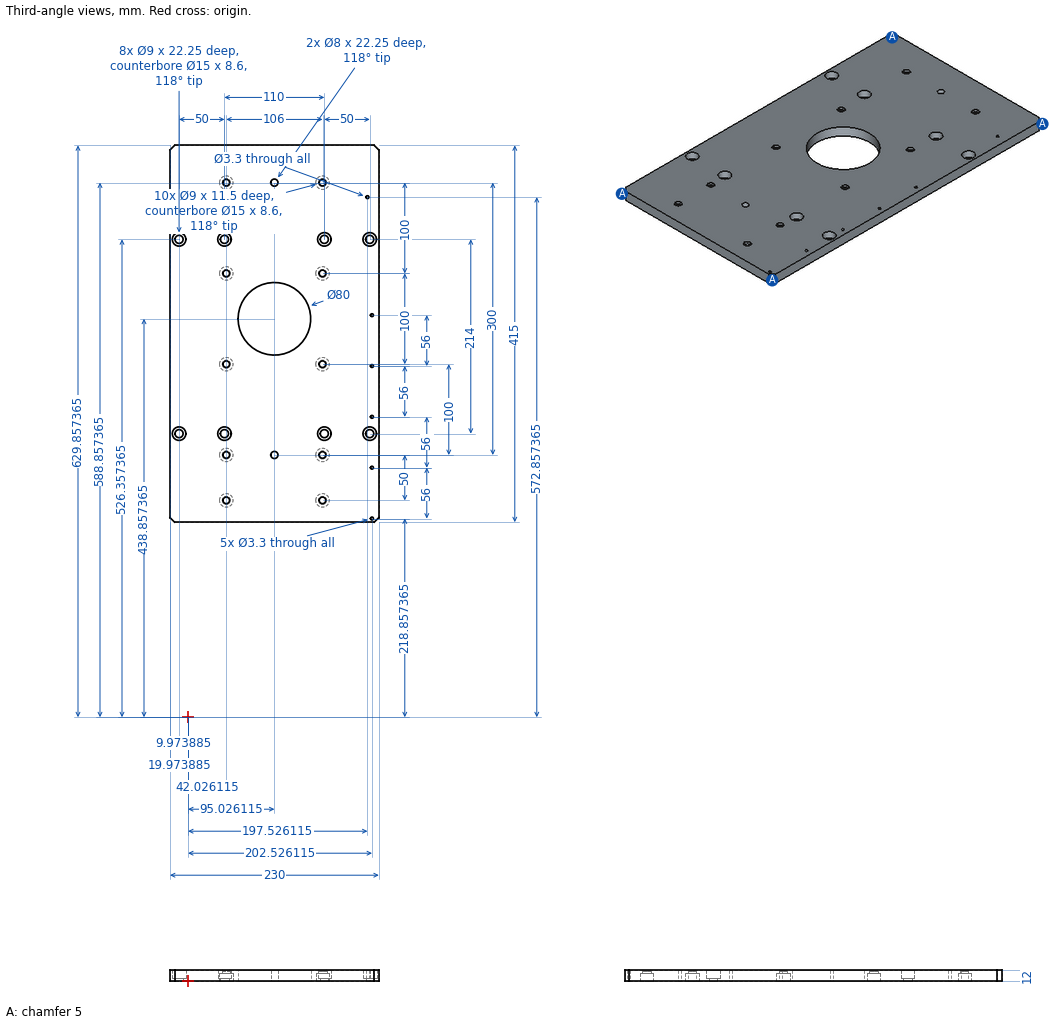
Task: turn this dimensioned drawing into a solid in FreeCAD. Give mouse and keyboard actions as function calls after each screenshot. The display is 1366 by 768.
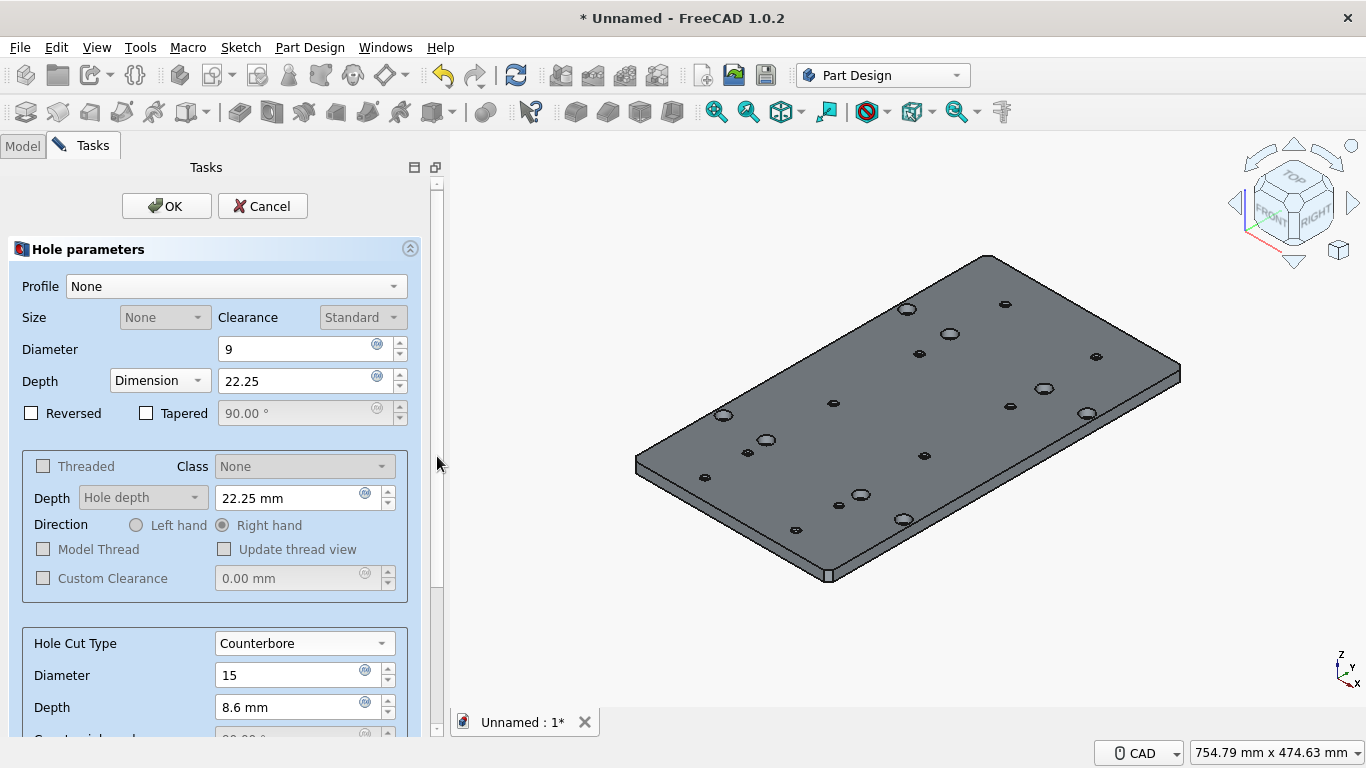
click(167, 206)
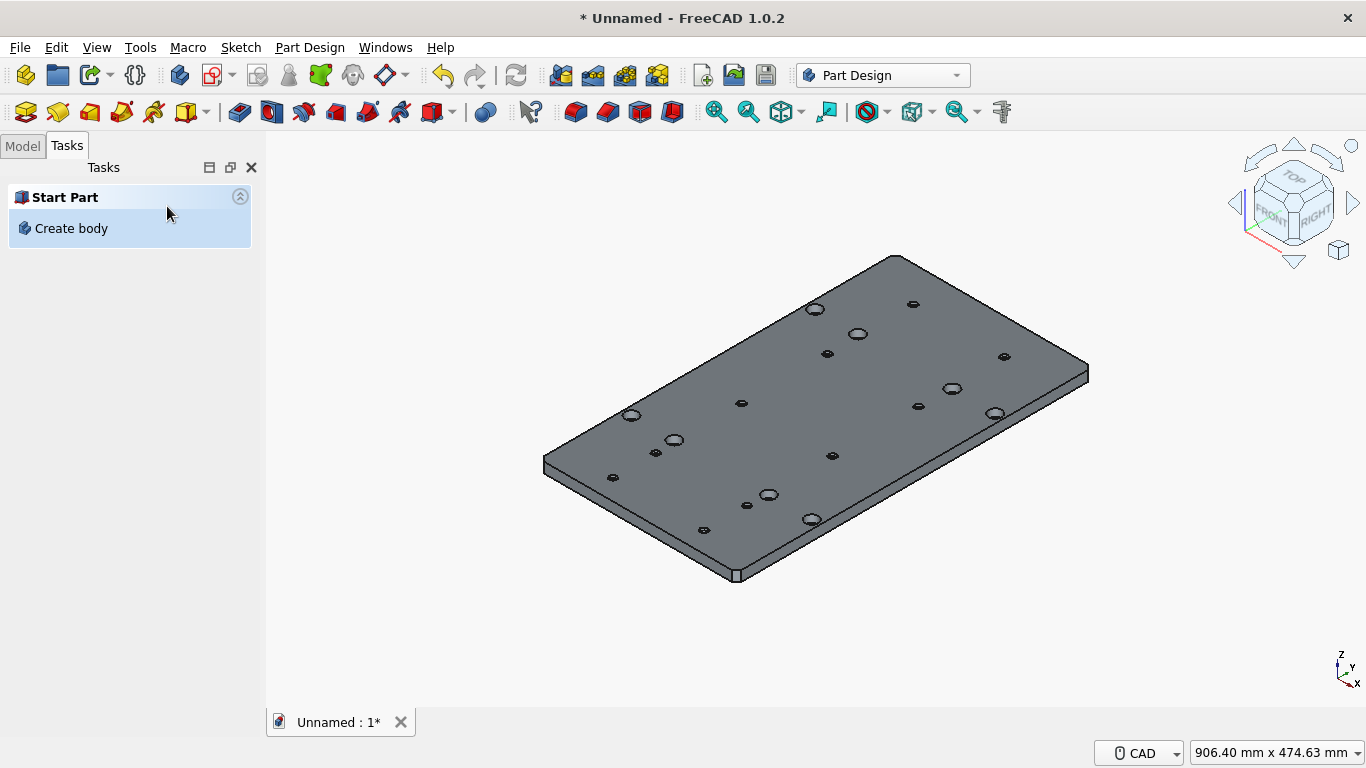
click(816, 412)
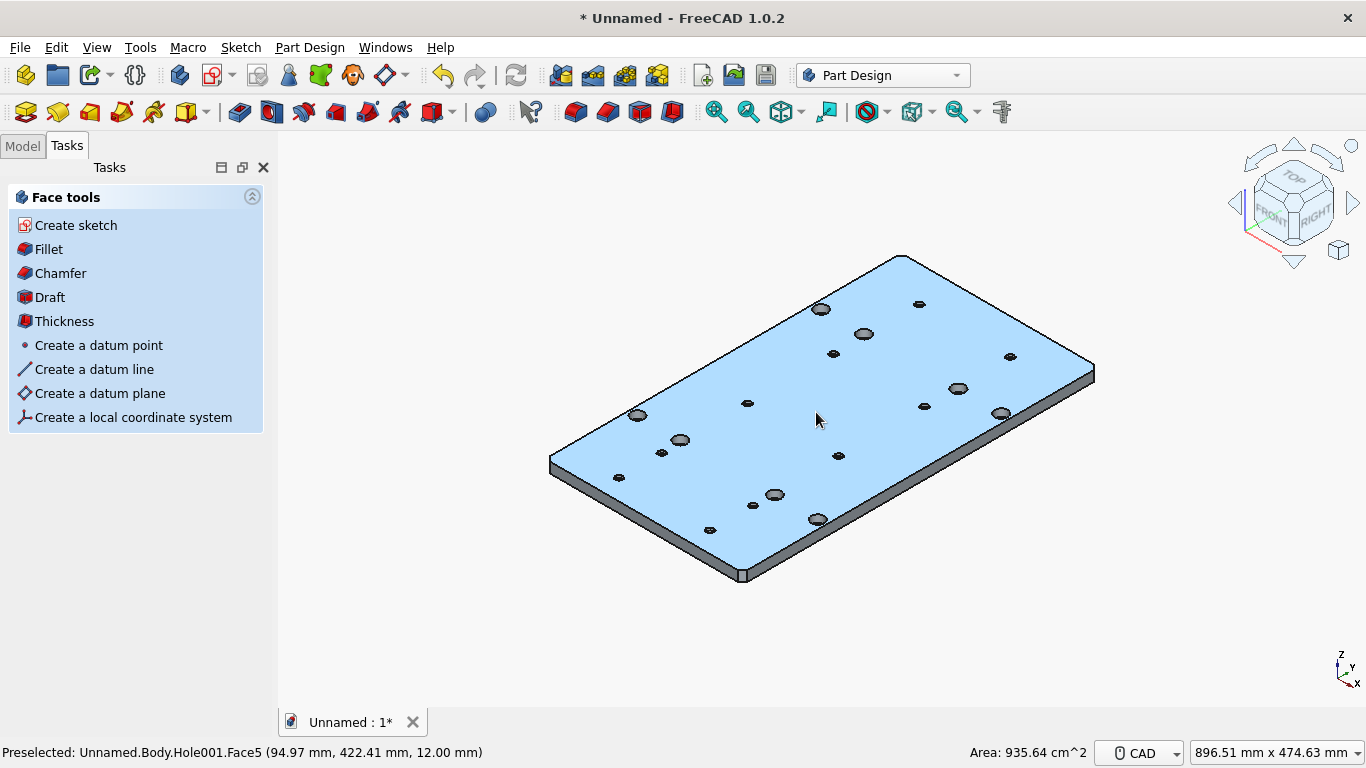
click(212, 76)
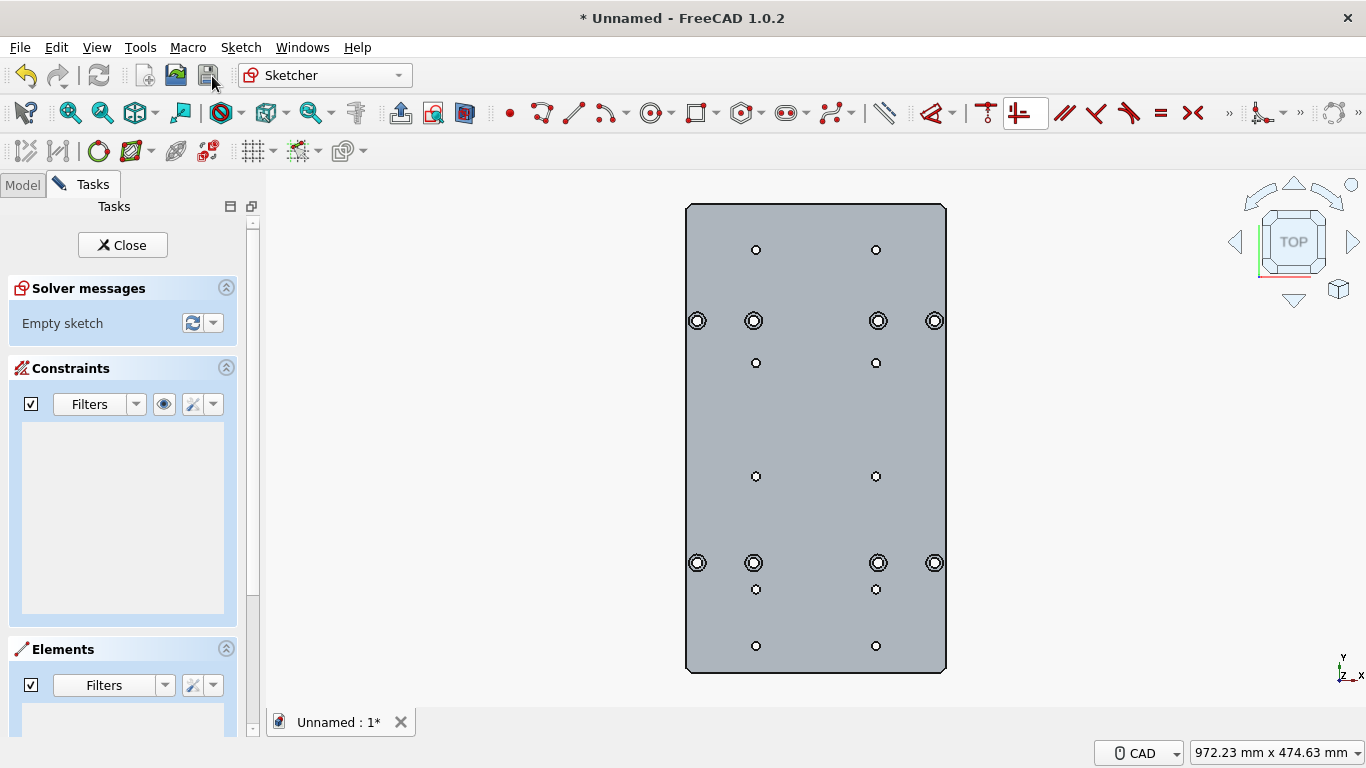
scroll(727, 265, down, 3)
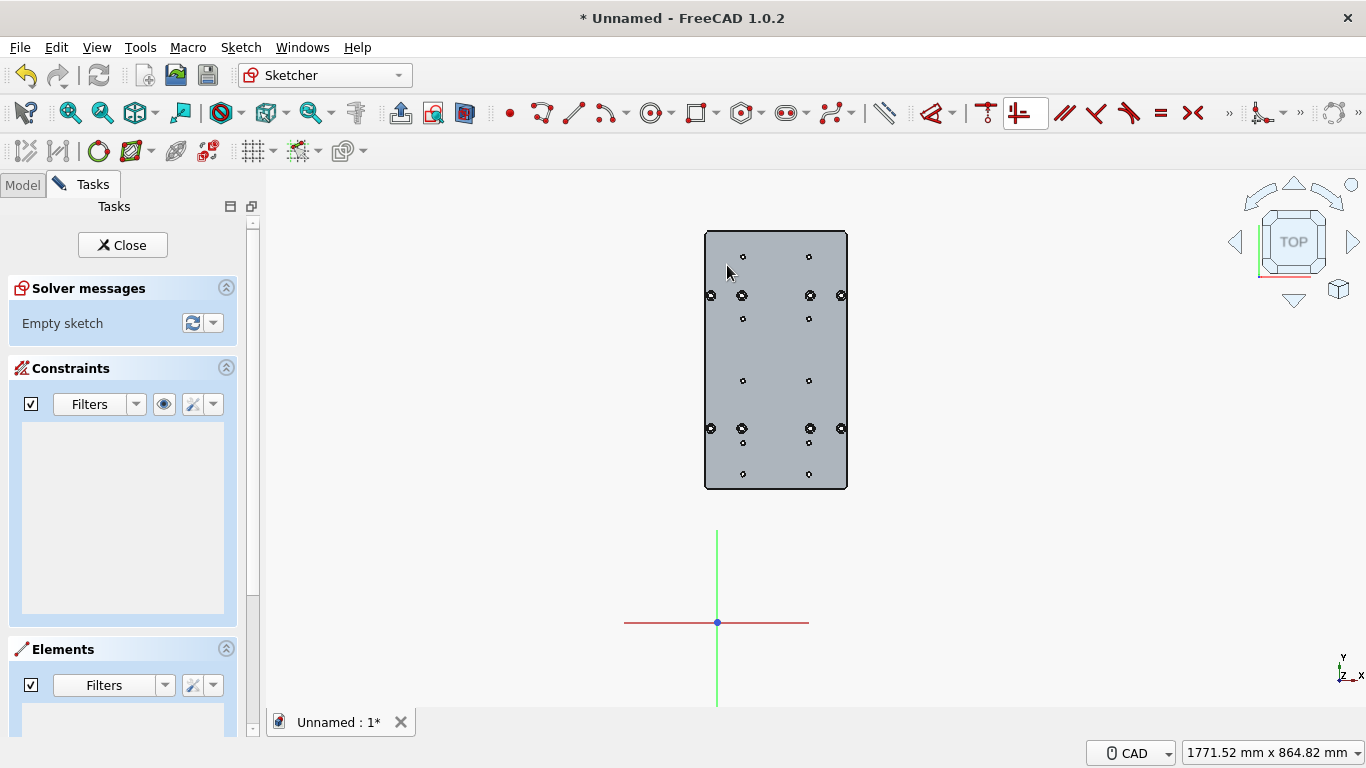
click(652, 114)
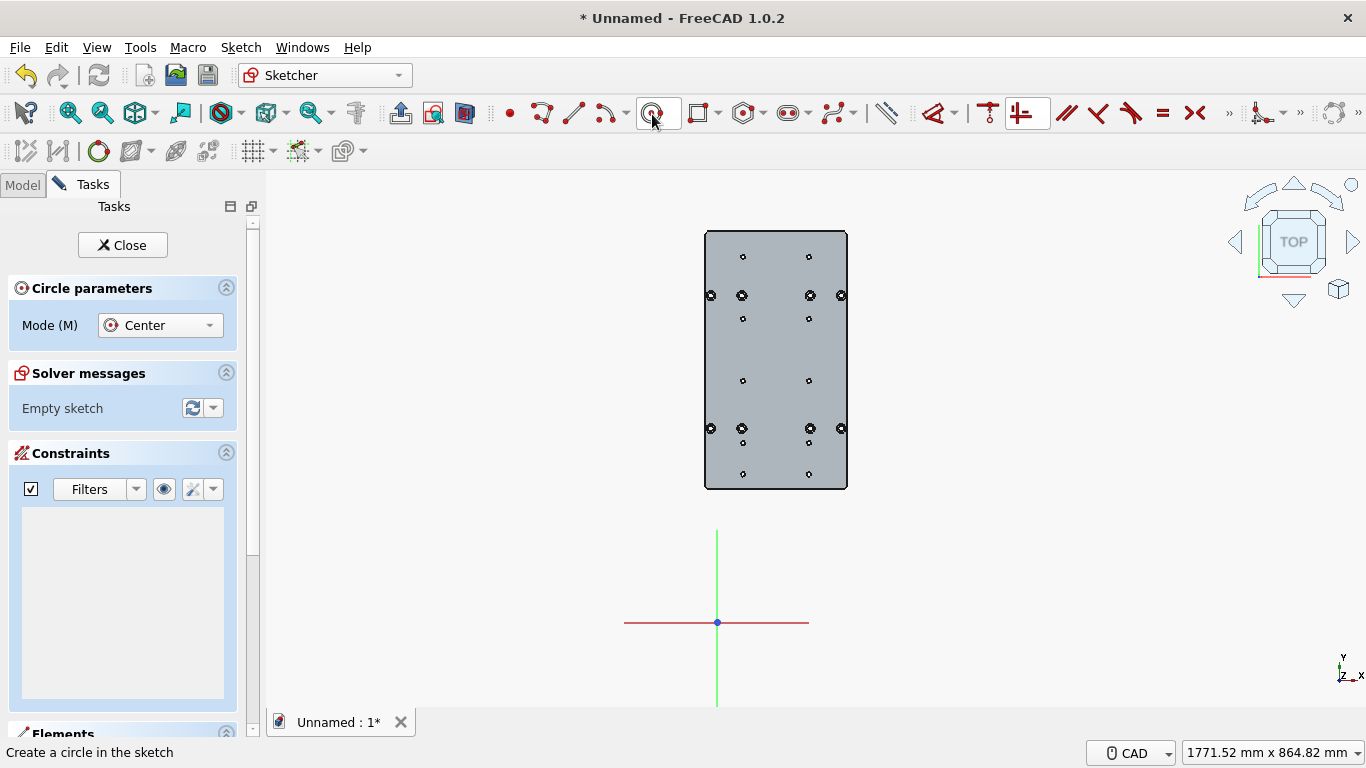
scroll(776, 257, up, 12)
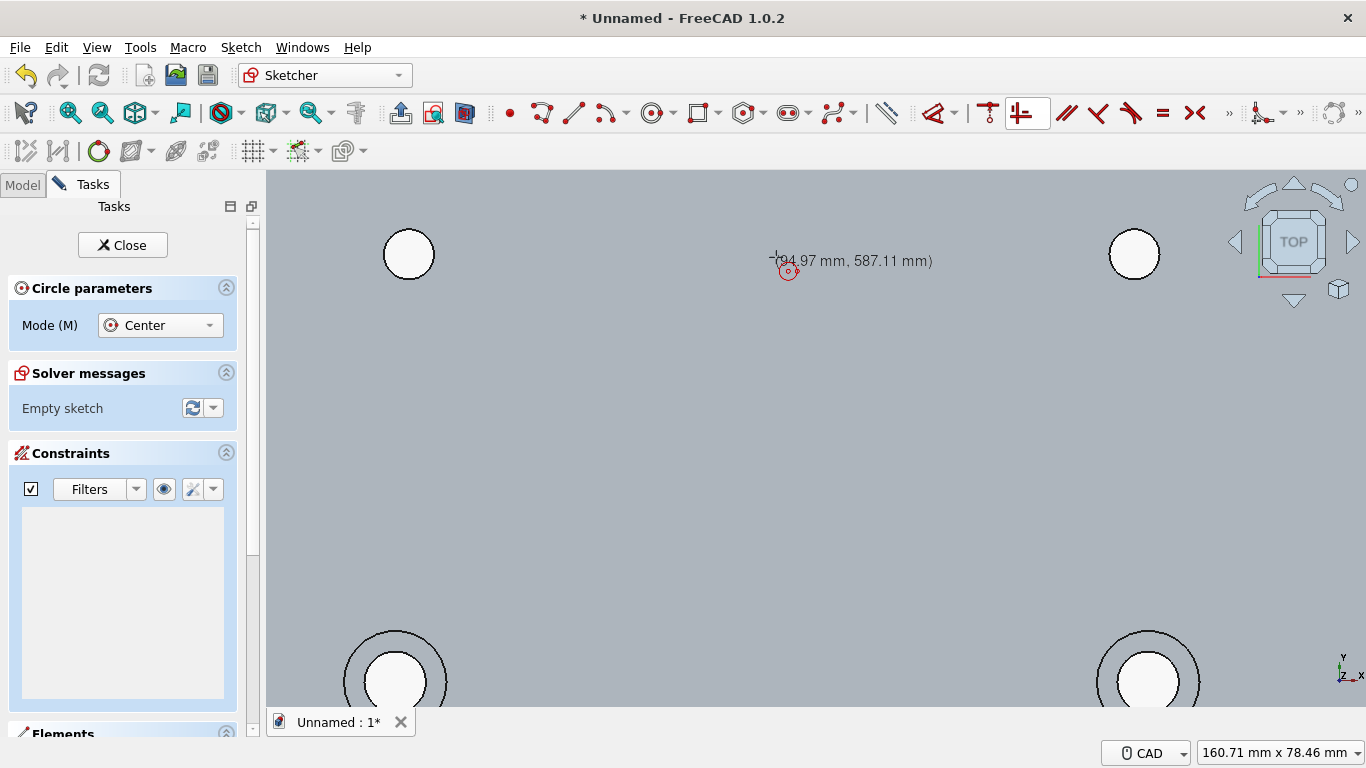
scroll(776, 257, down, 12)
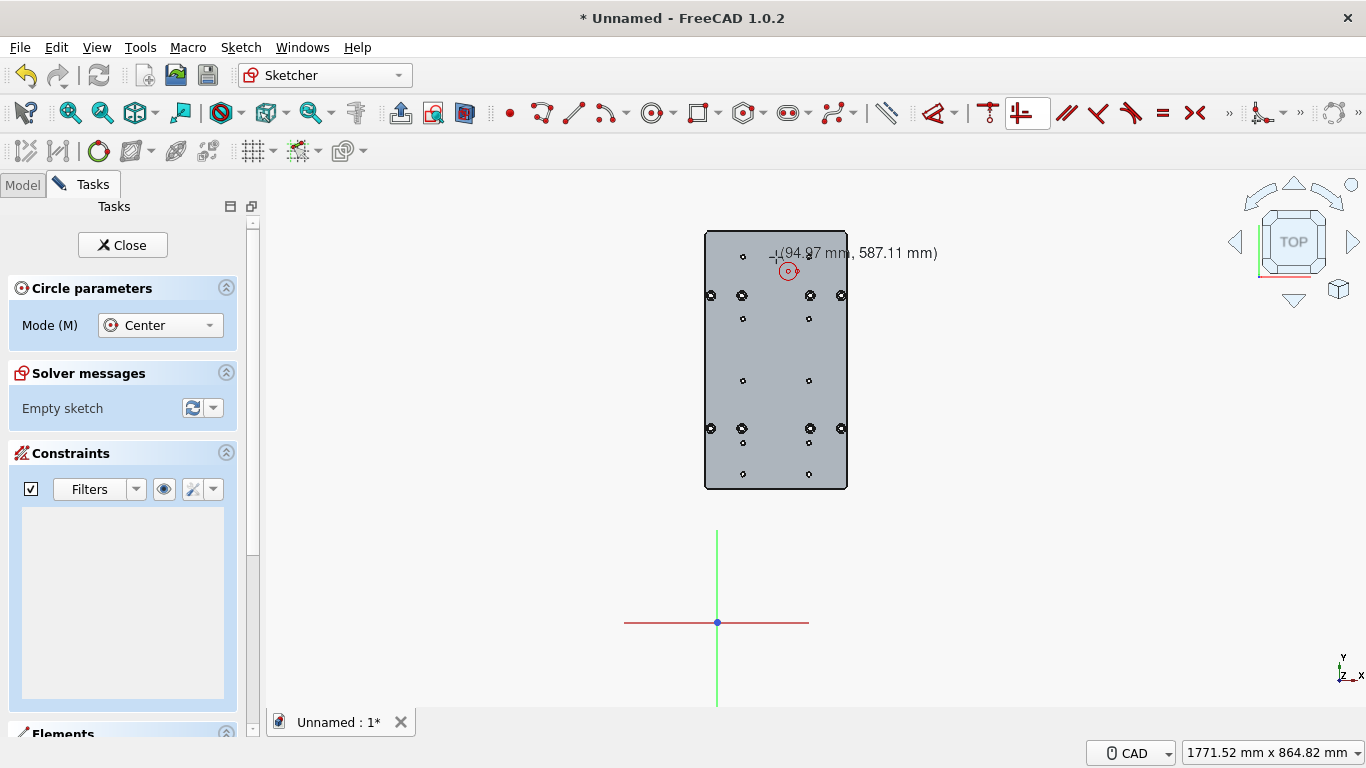
click(776, 257)
move(778, 255)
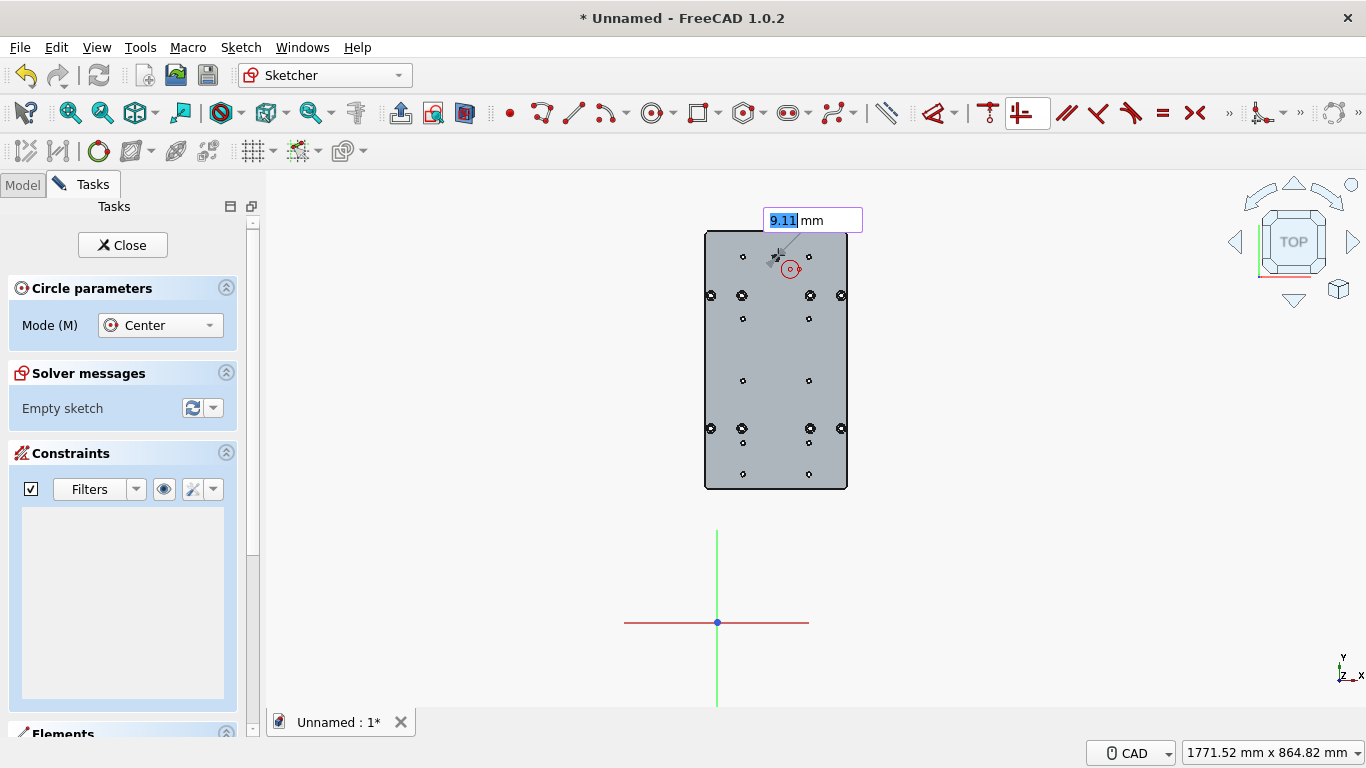
text(8)
key(Return)